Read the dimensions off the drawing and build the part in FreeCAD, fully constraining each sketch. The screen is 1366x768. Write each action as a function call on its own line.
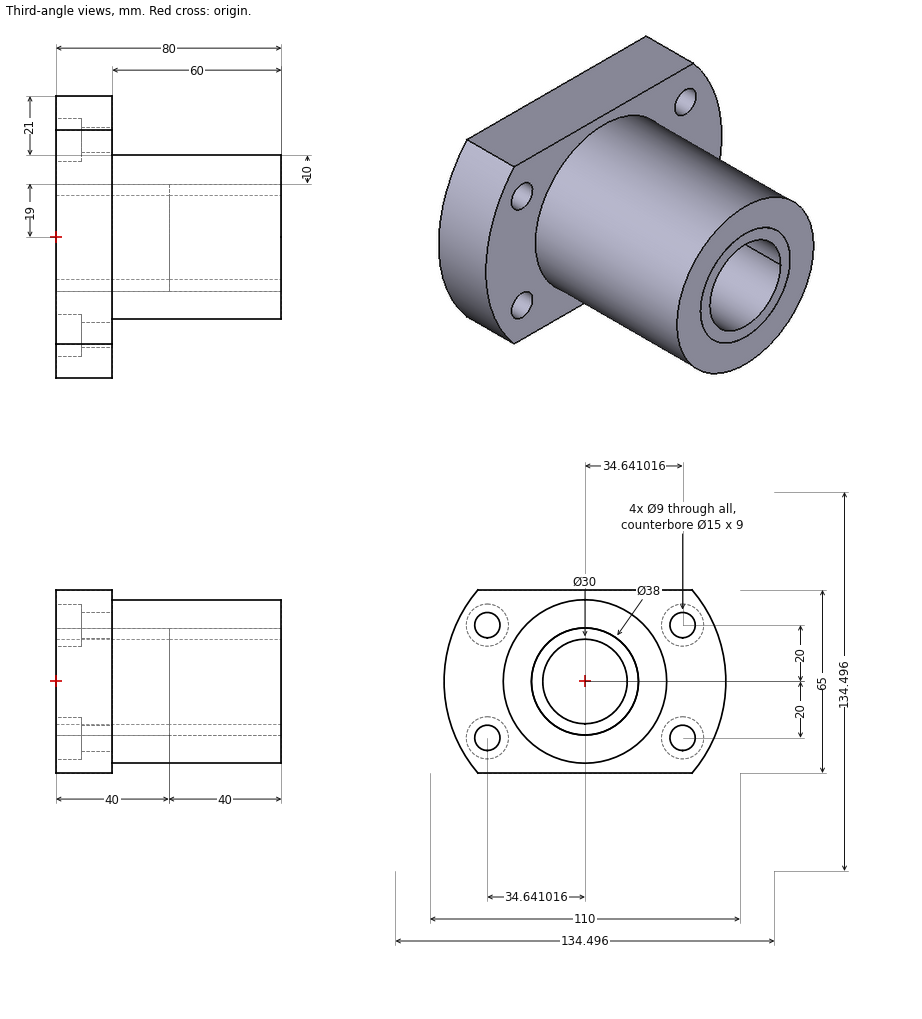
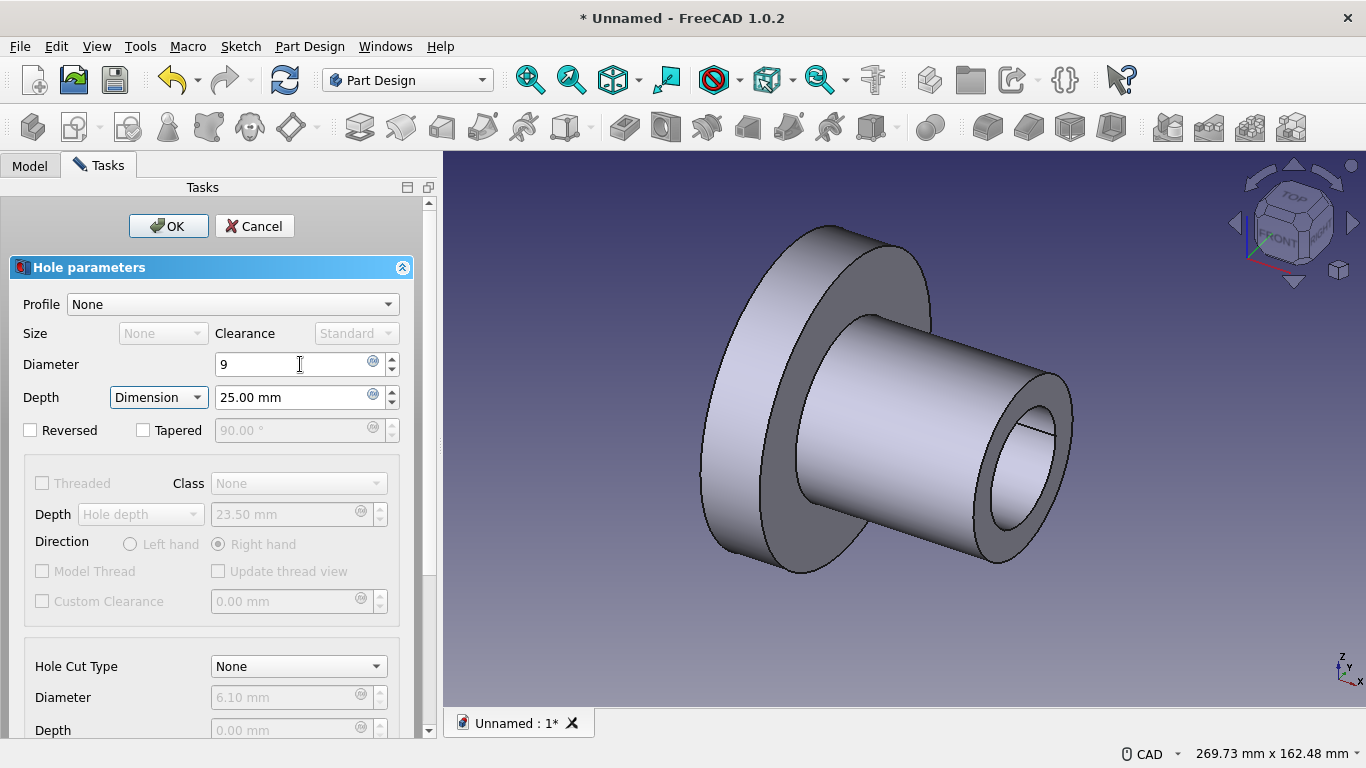
click(160, 398)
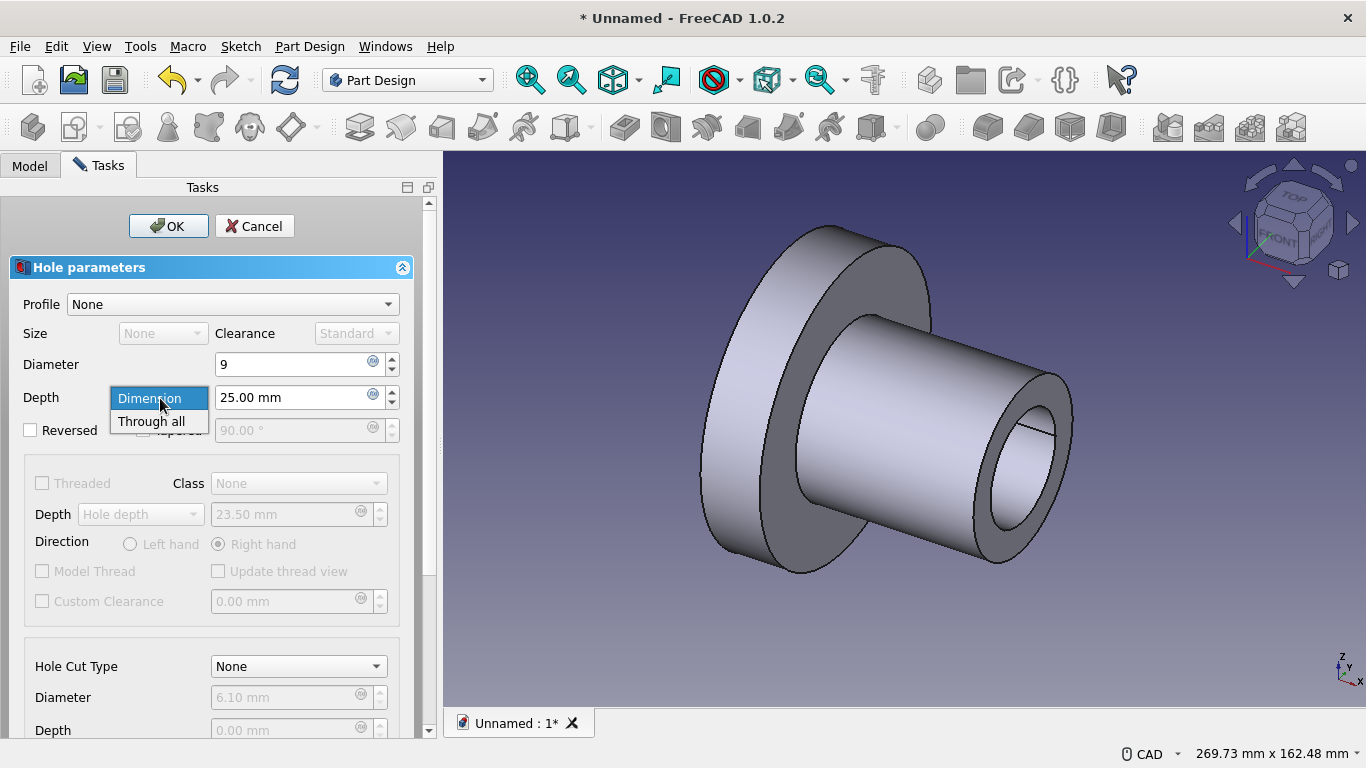
click(158, 422)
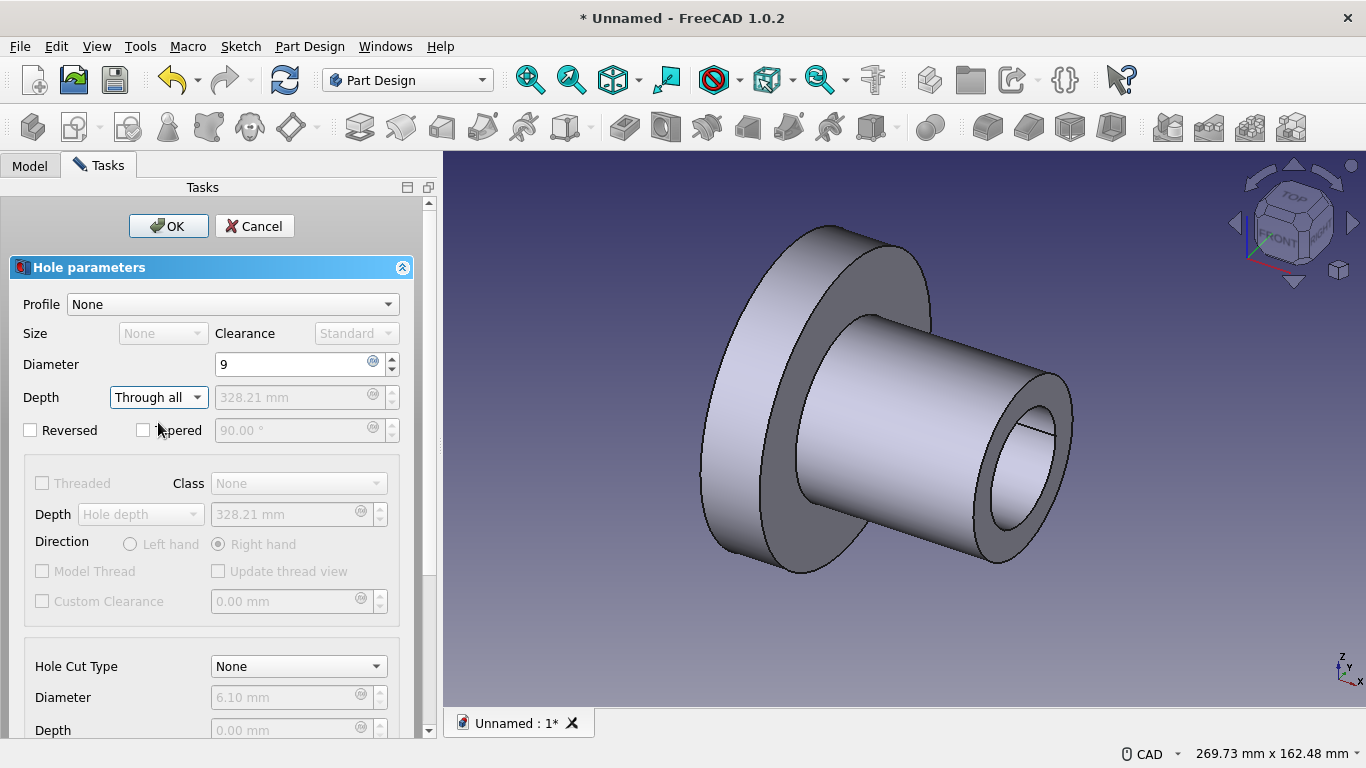
click(31, 430)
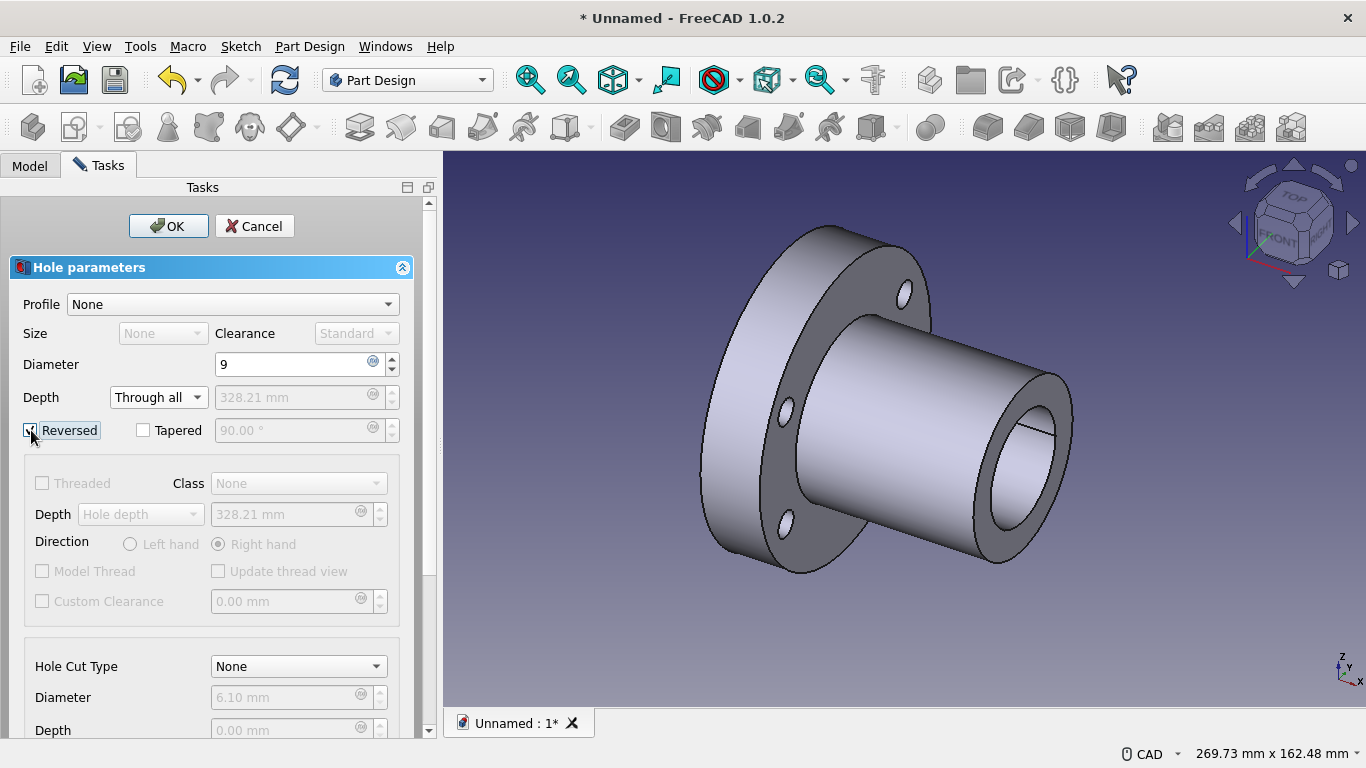
click(300, 666)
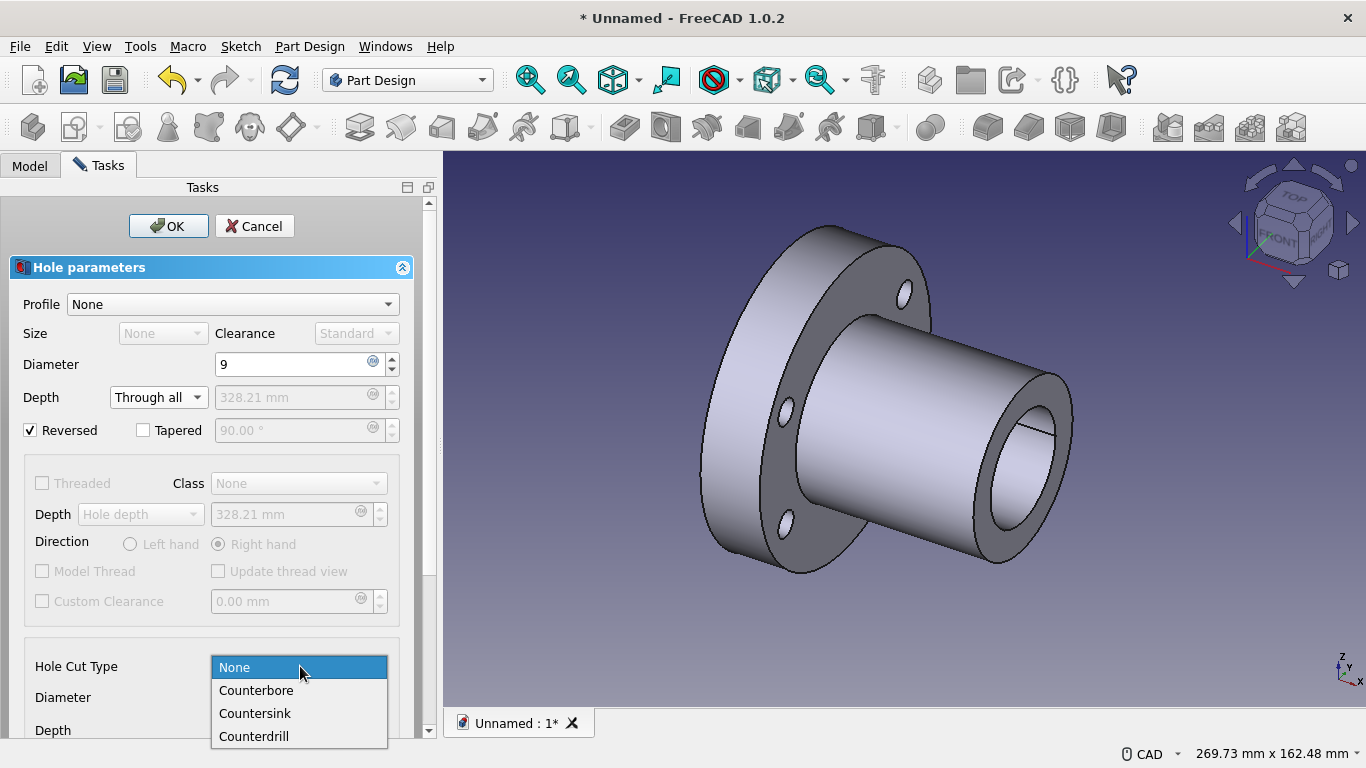
click(298, 690)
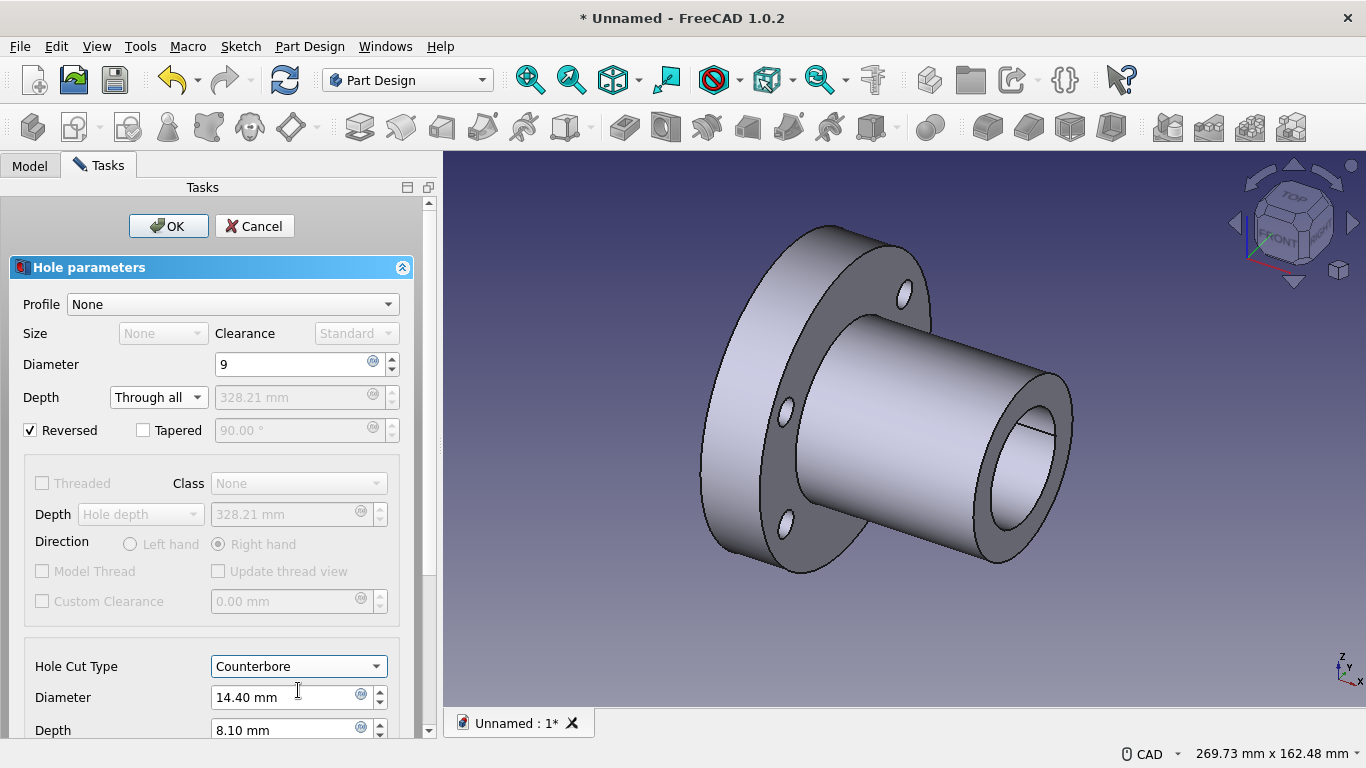
triple_click(292, 698)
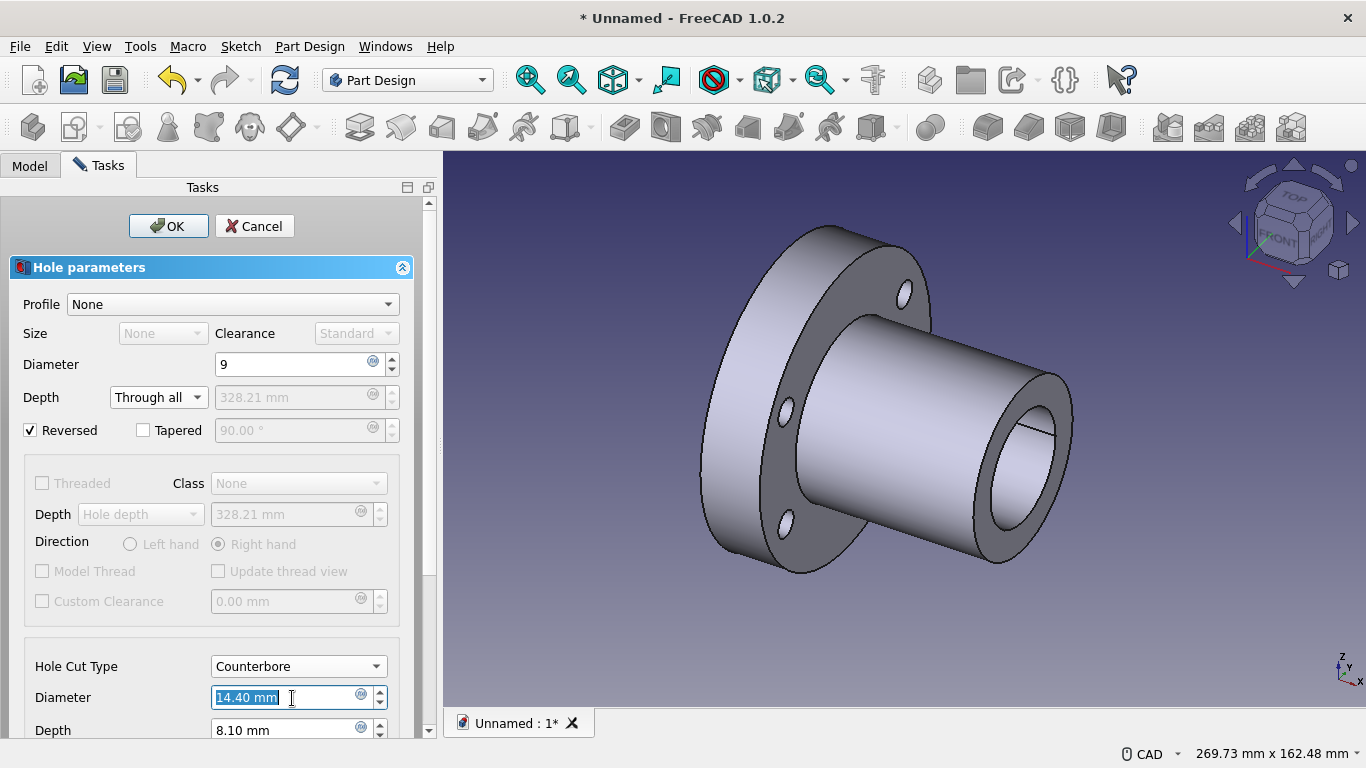
text(15)
key(Tab)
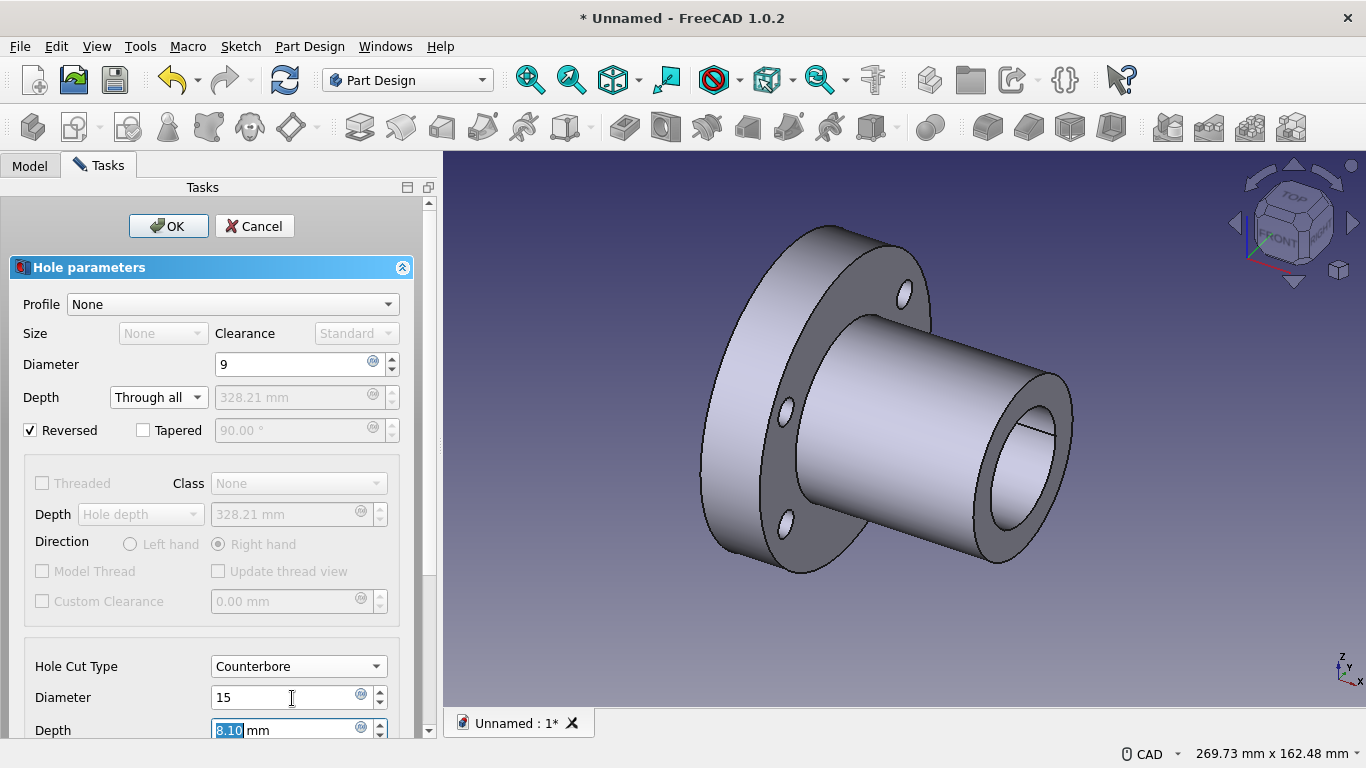
scroll(429, 468, down, 2)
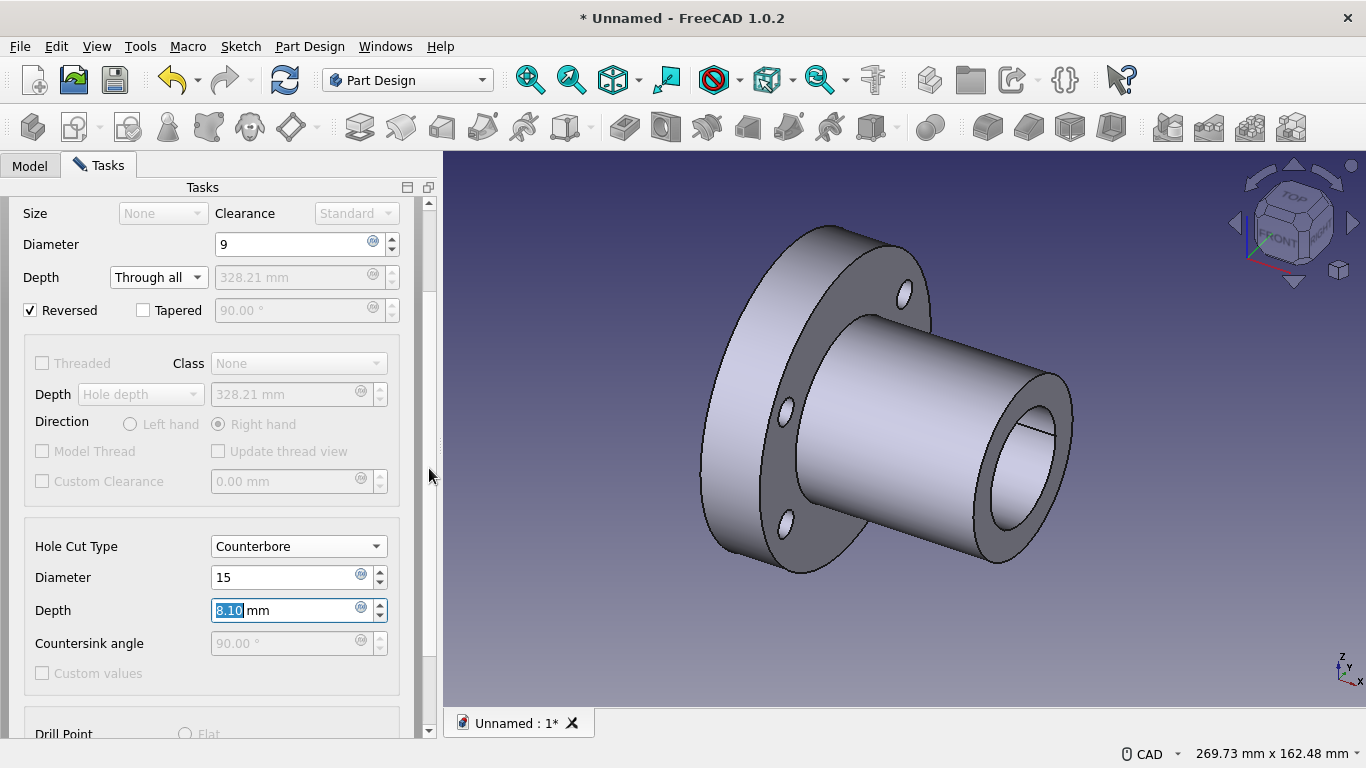
text(9)
key(Tab)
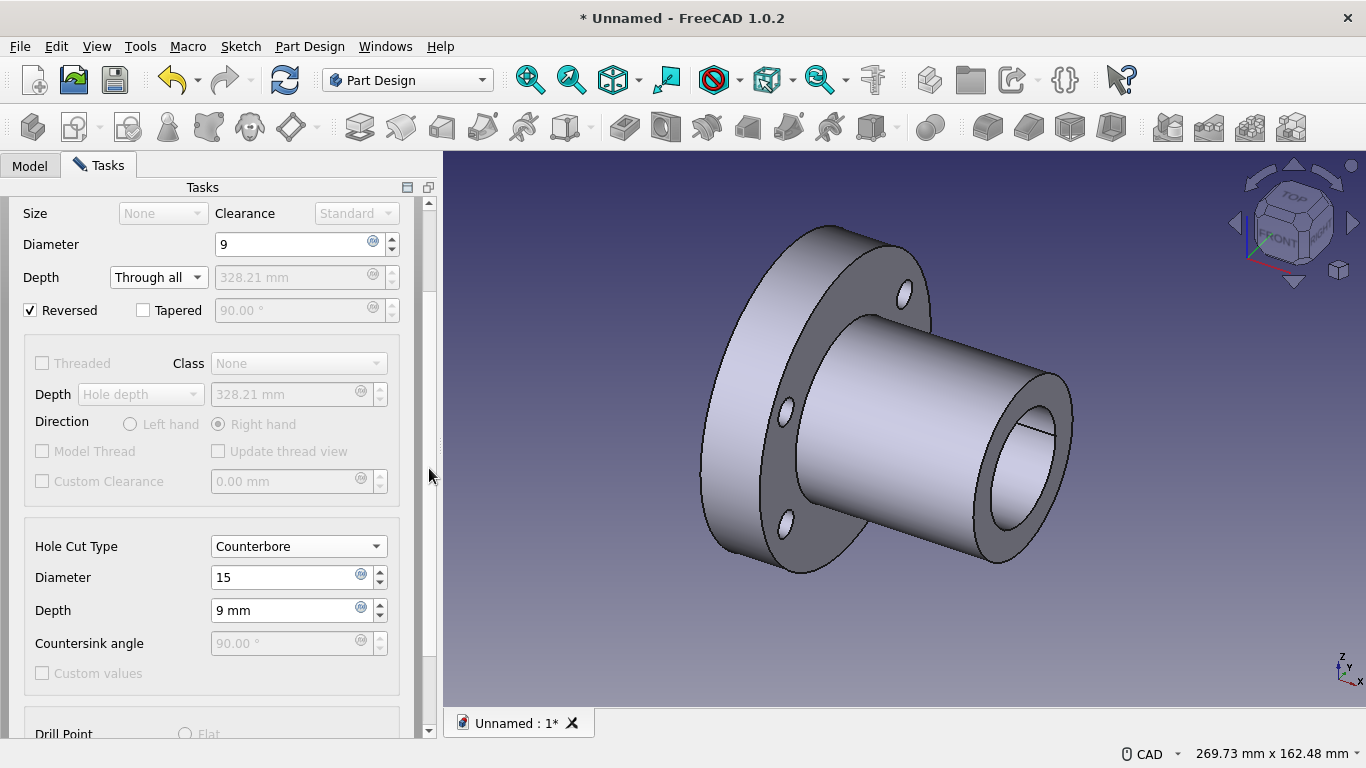
scroll(429, 468, up, 3)